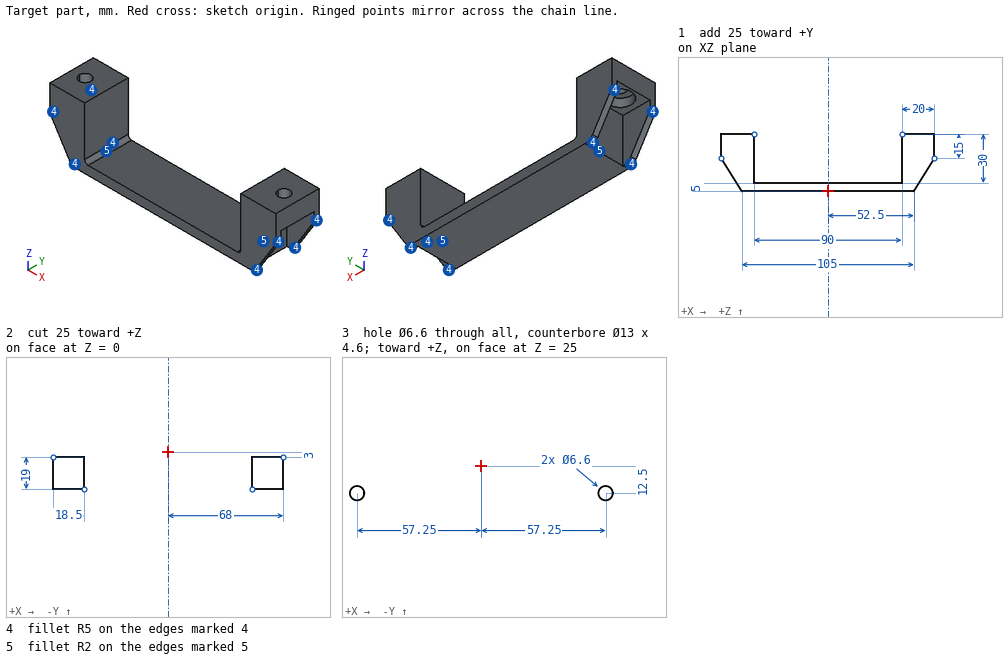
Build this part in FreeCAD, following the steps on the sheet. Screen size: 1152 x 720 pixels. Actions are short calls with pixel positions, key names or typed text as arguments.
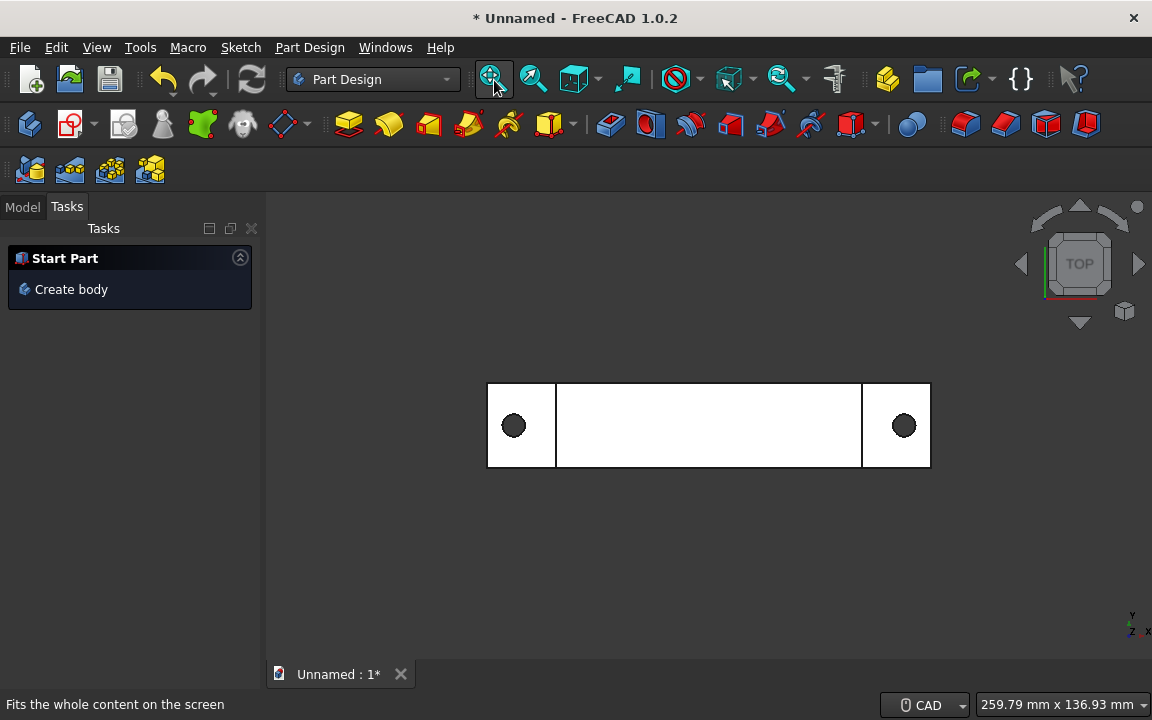
key(1)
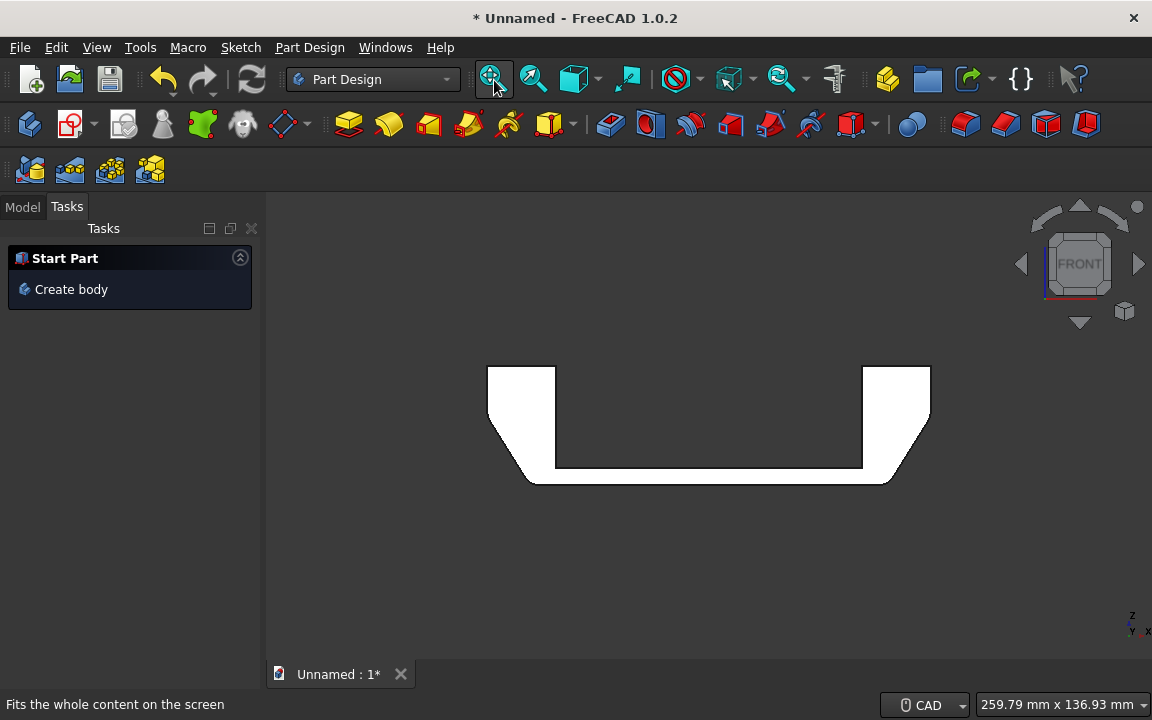
key(3)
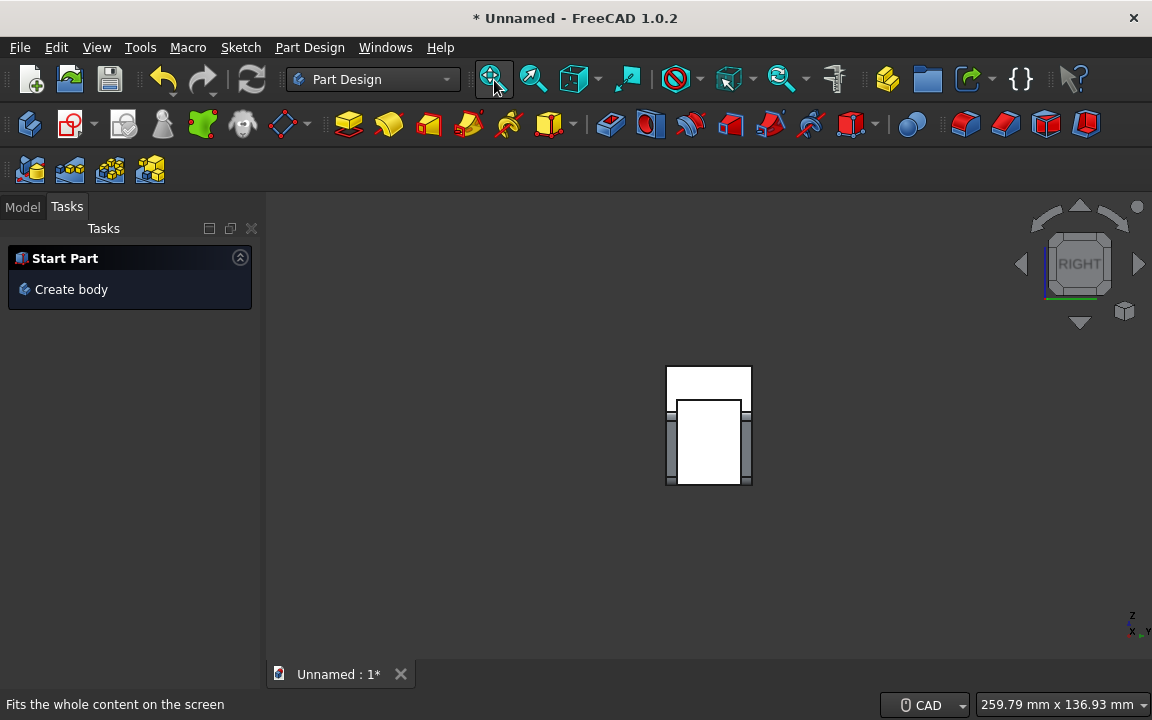
click(494, 80)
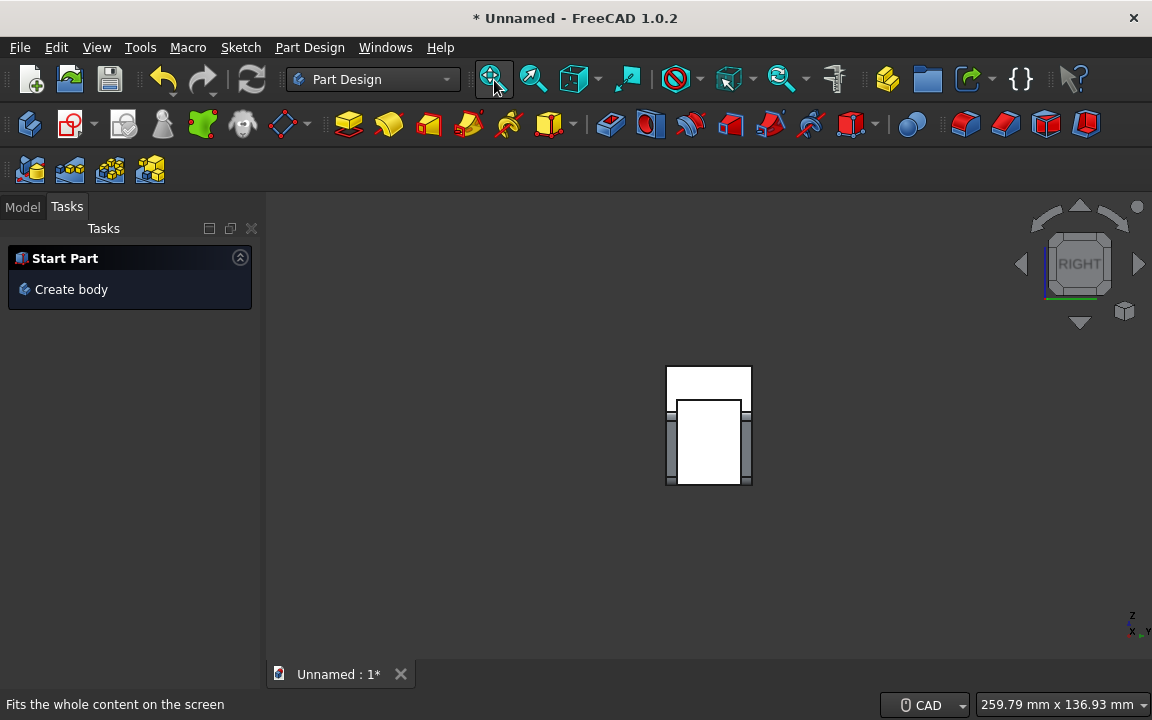
key(5)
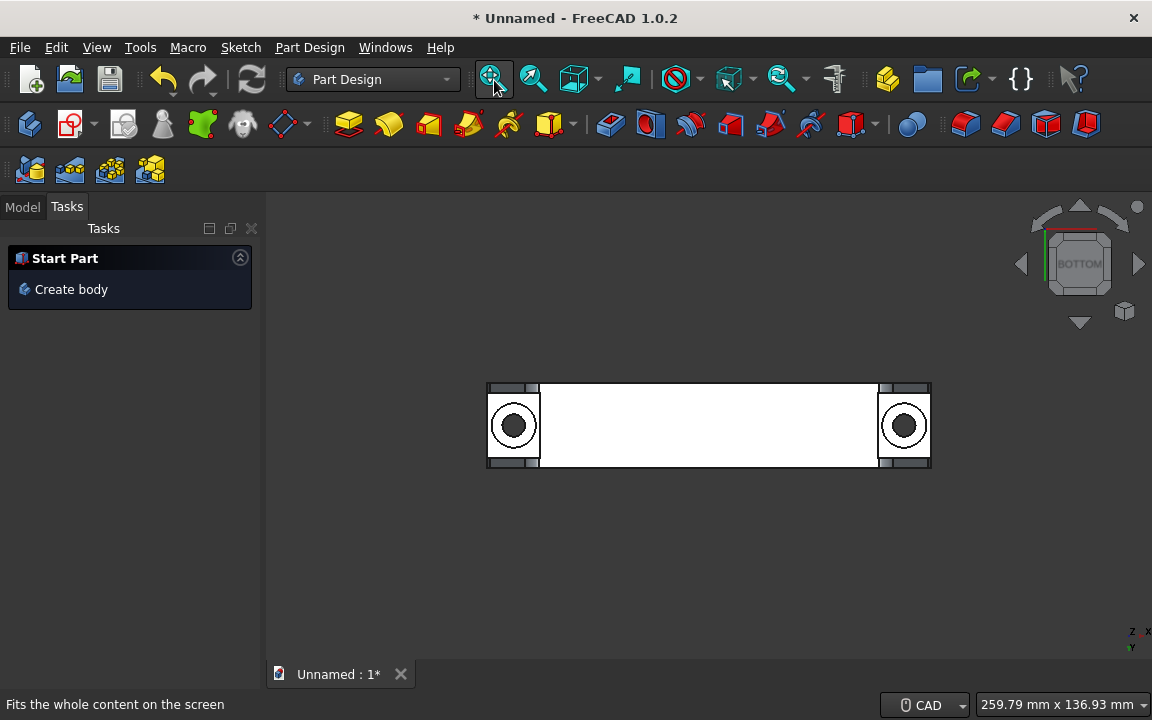
key(4)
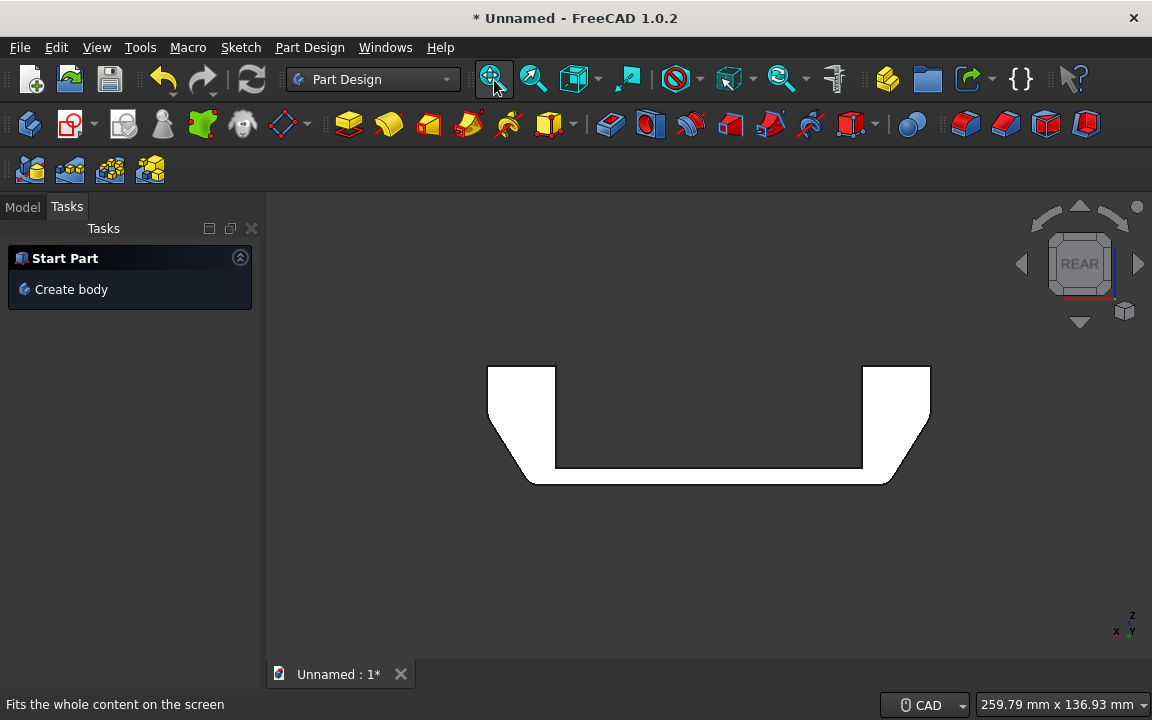
key(6)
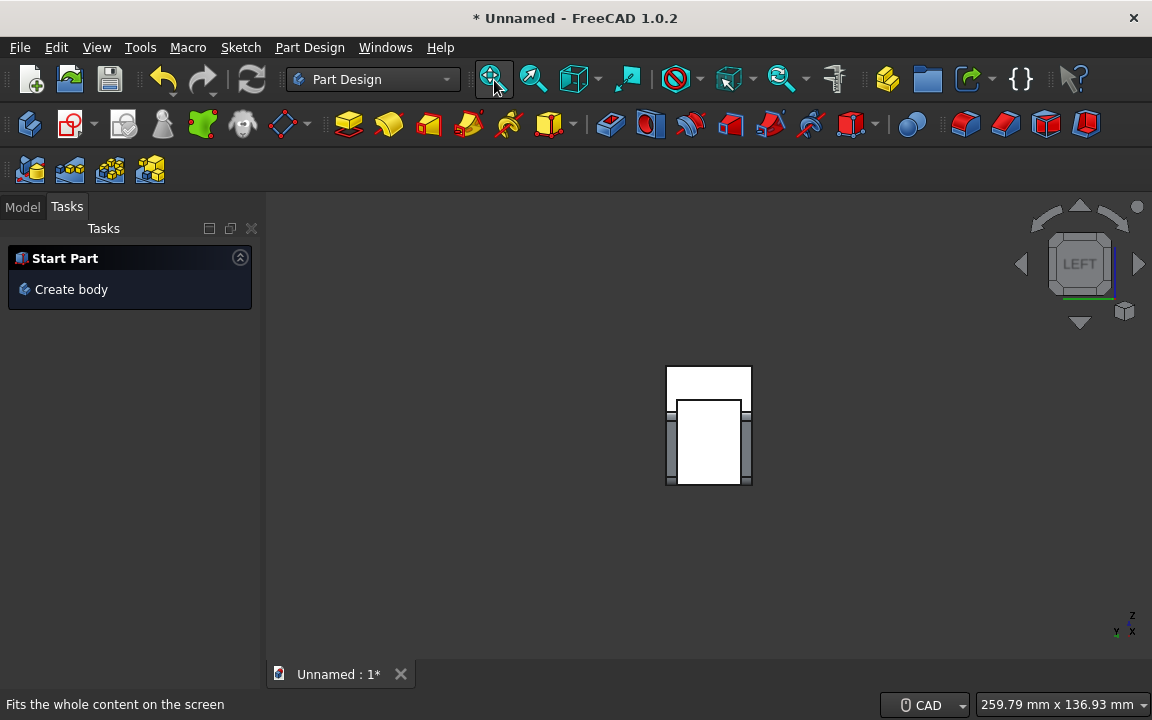
click(494, 80)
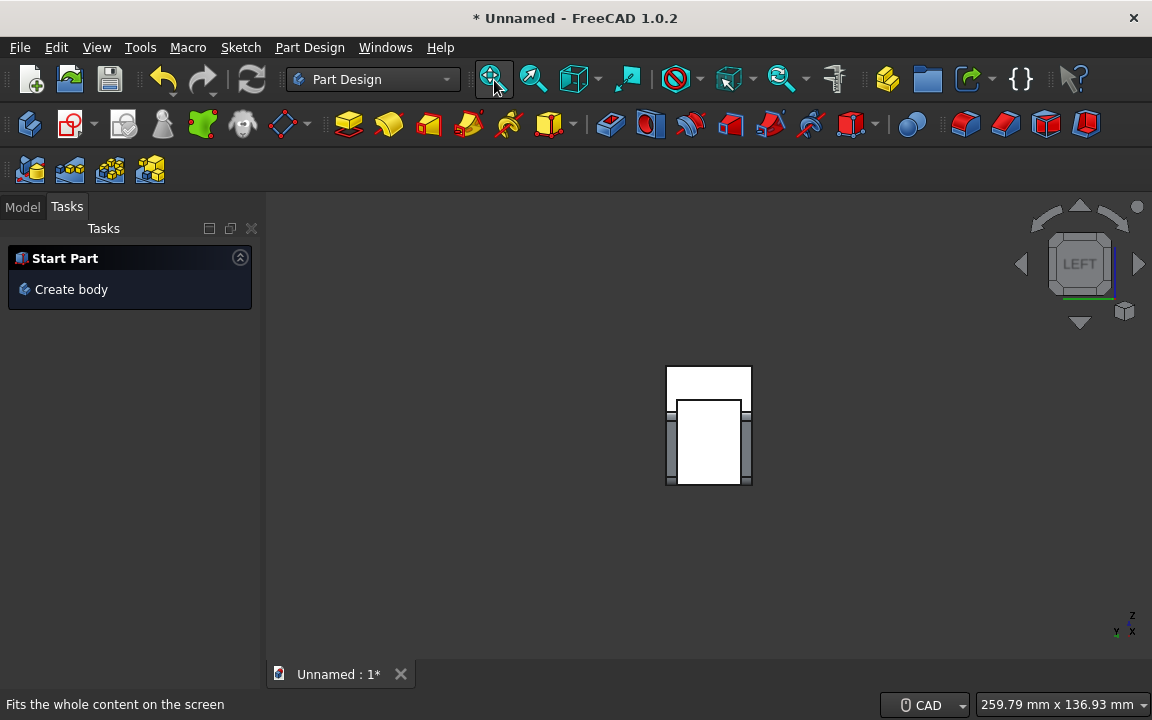
key(v)
key(3)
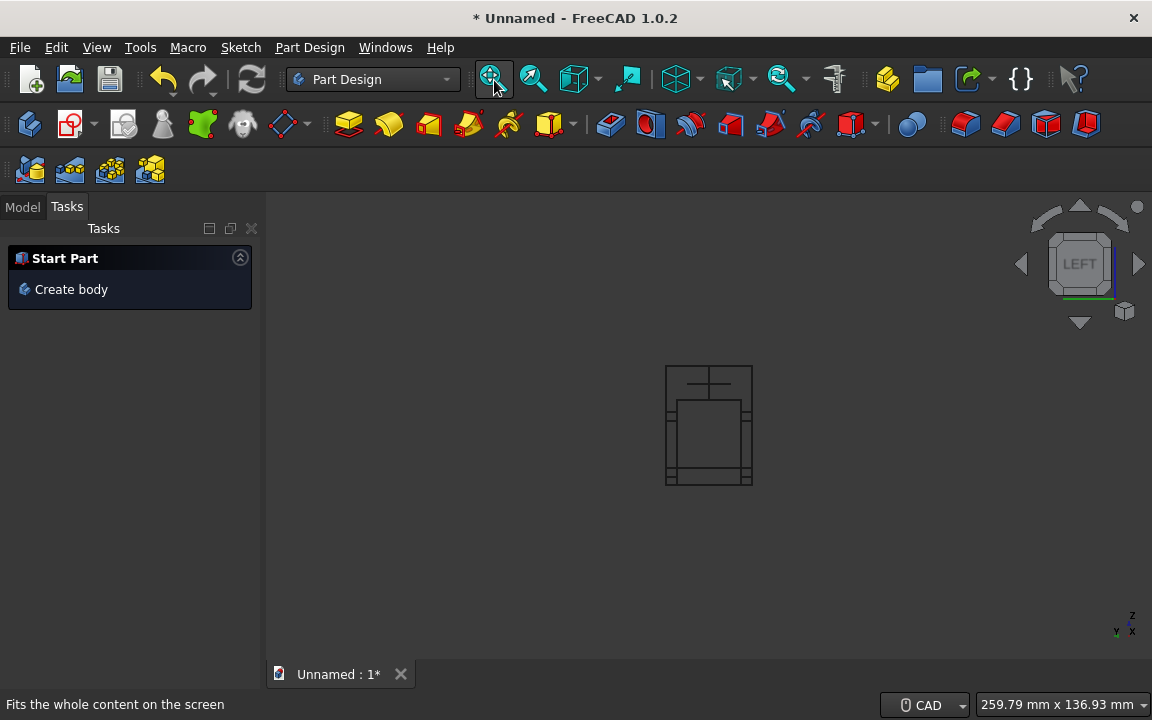
key(0)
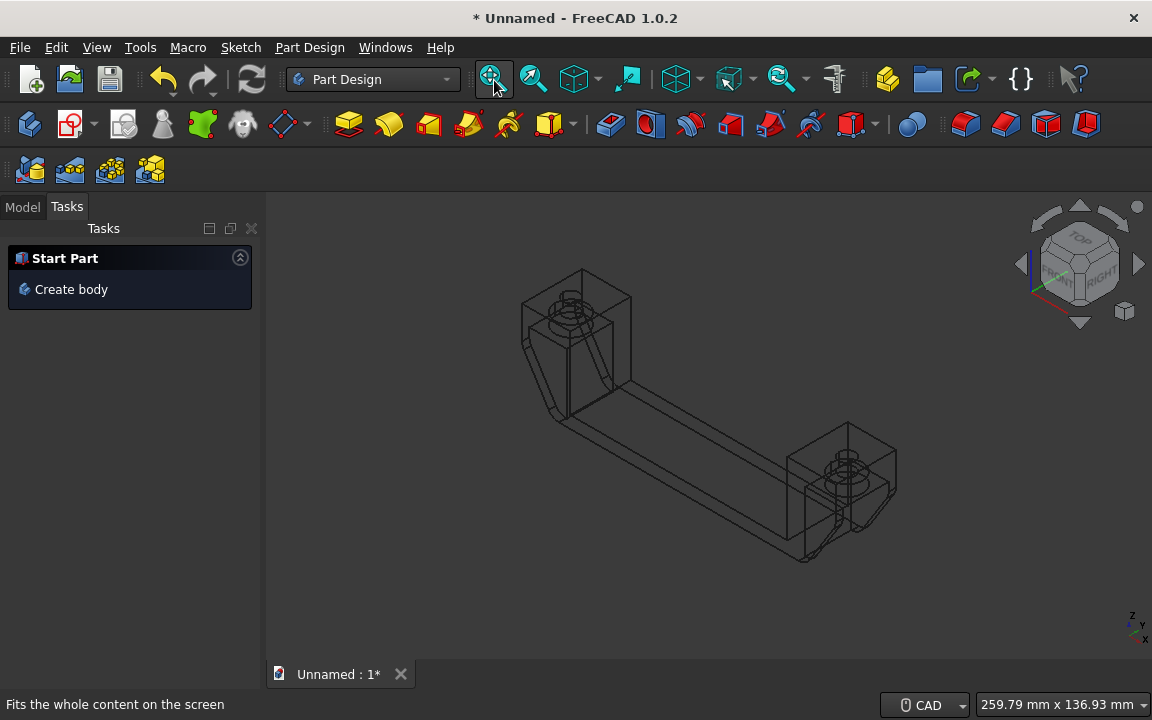
click(818, 522)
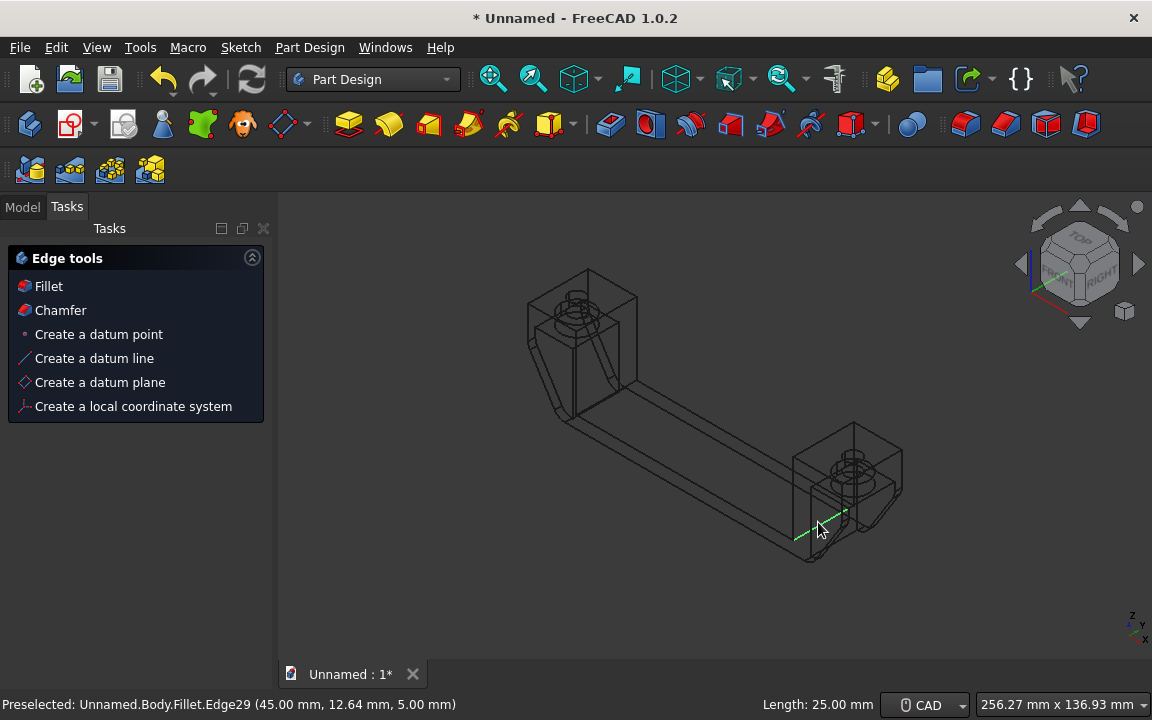
click(606, 397, ctrl)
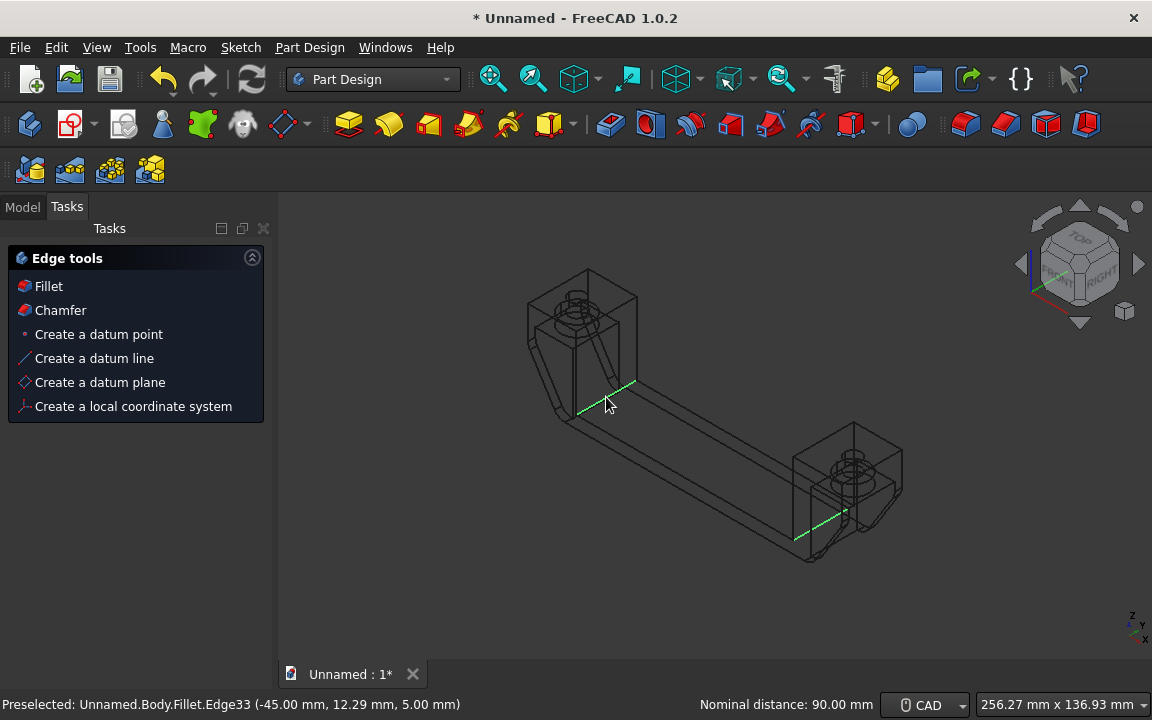
key(v)
key(1)